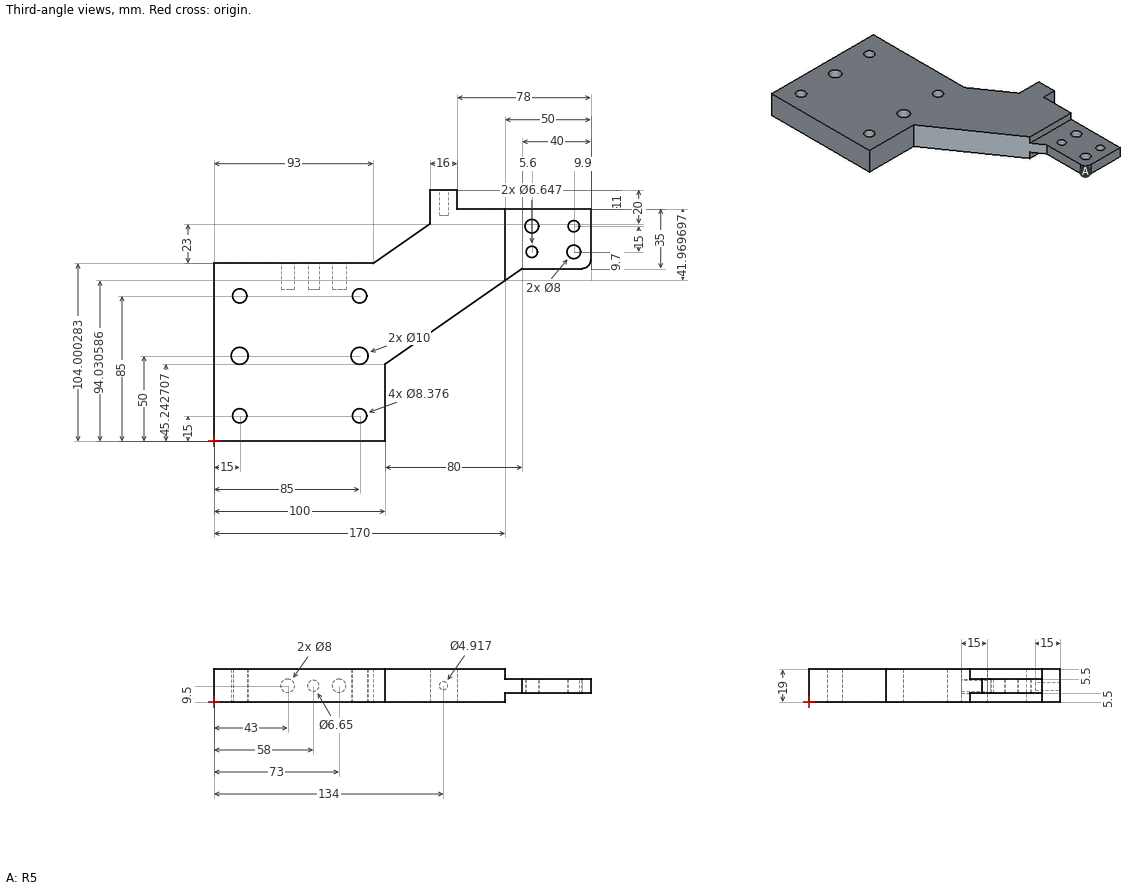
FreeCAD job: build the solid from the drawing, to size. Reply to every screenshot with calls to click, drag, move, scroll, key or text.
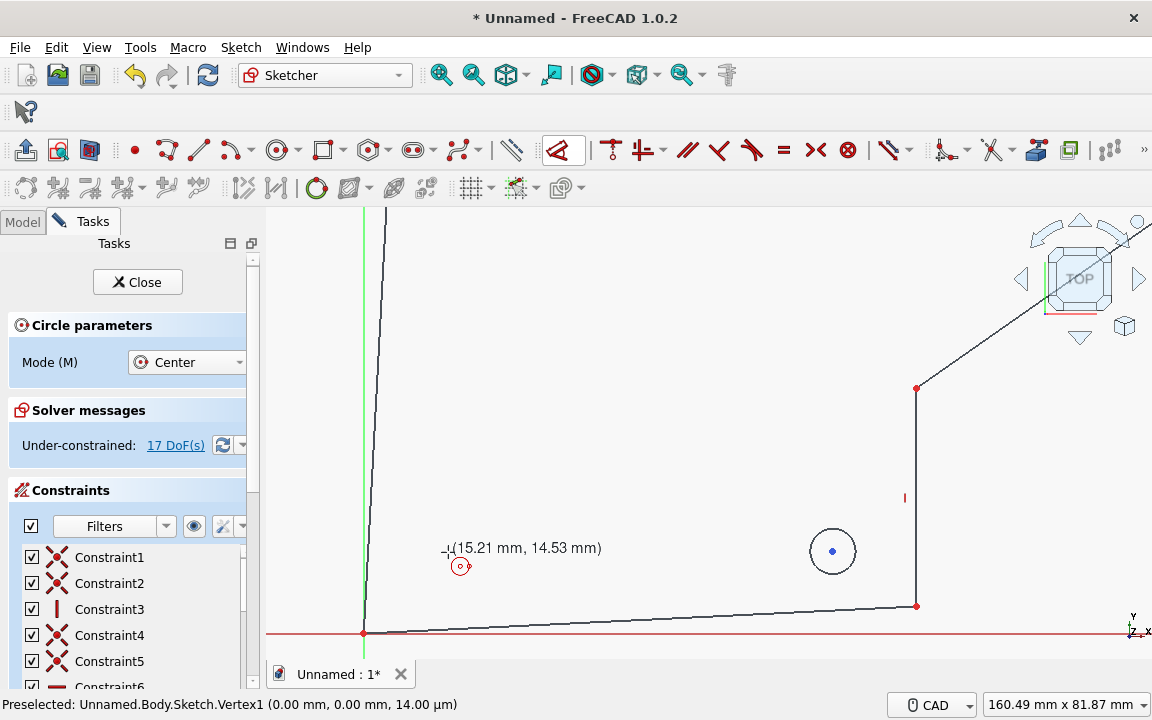
click(447, 551)
click(463, 534)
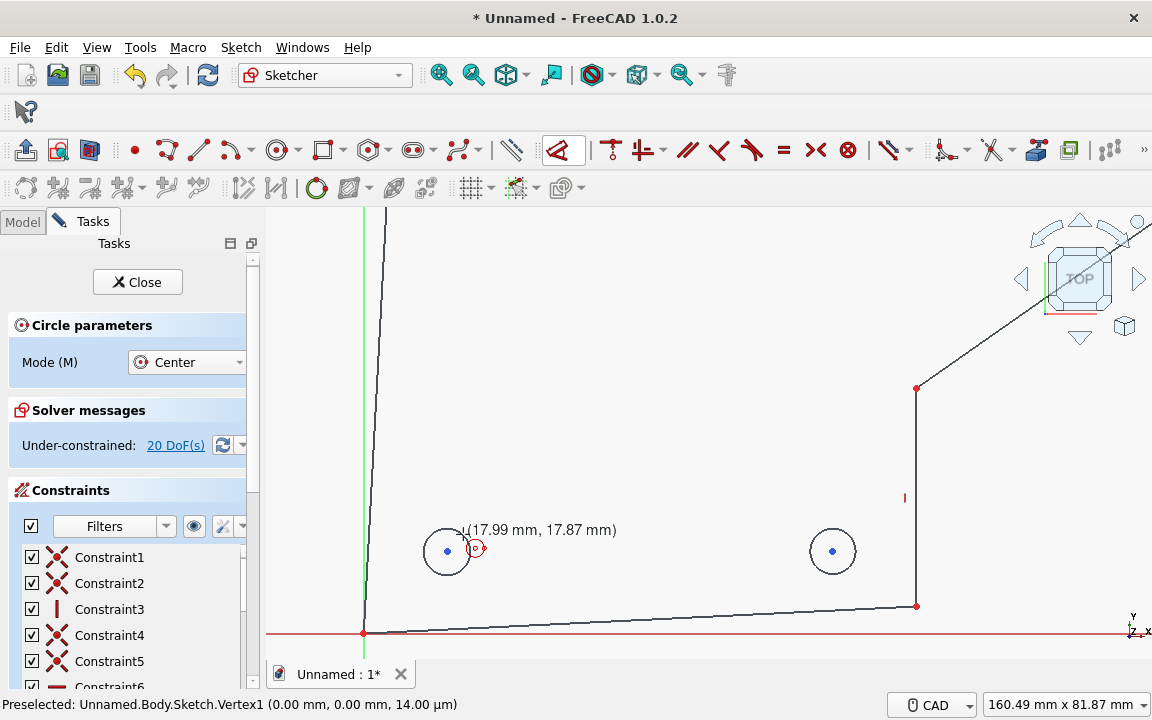
click(833, 358)
click(852, 338)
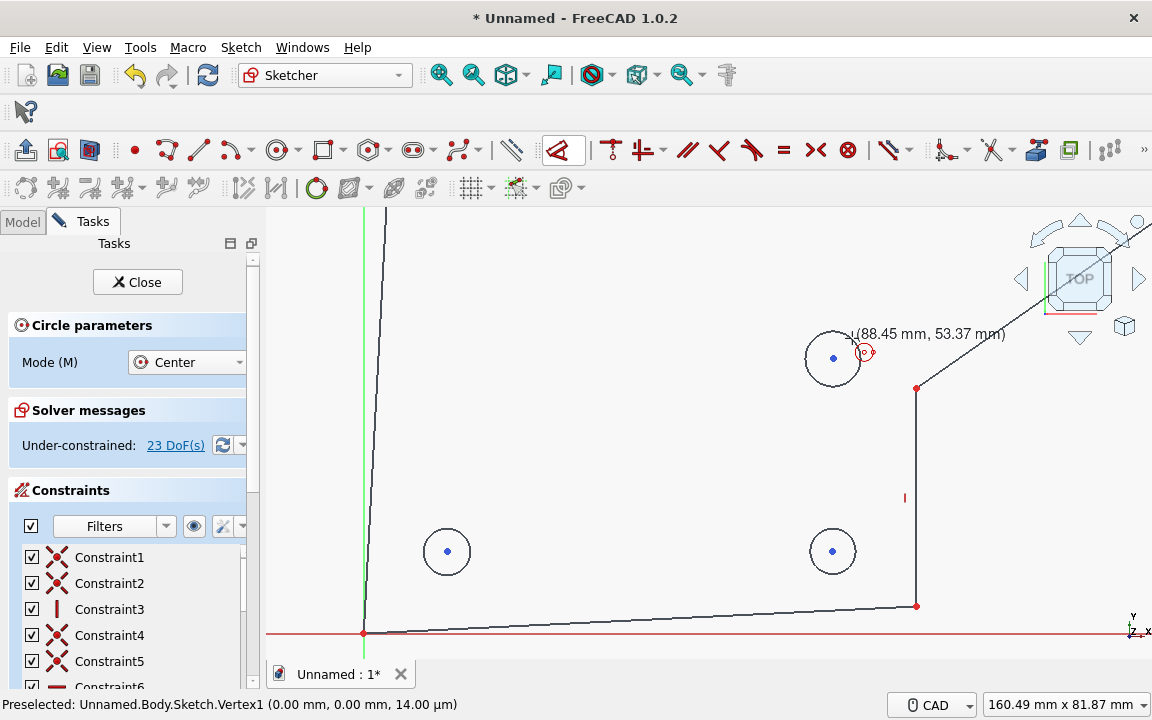
click(447, 358)
click(466, 338)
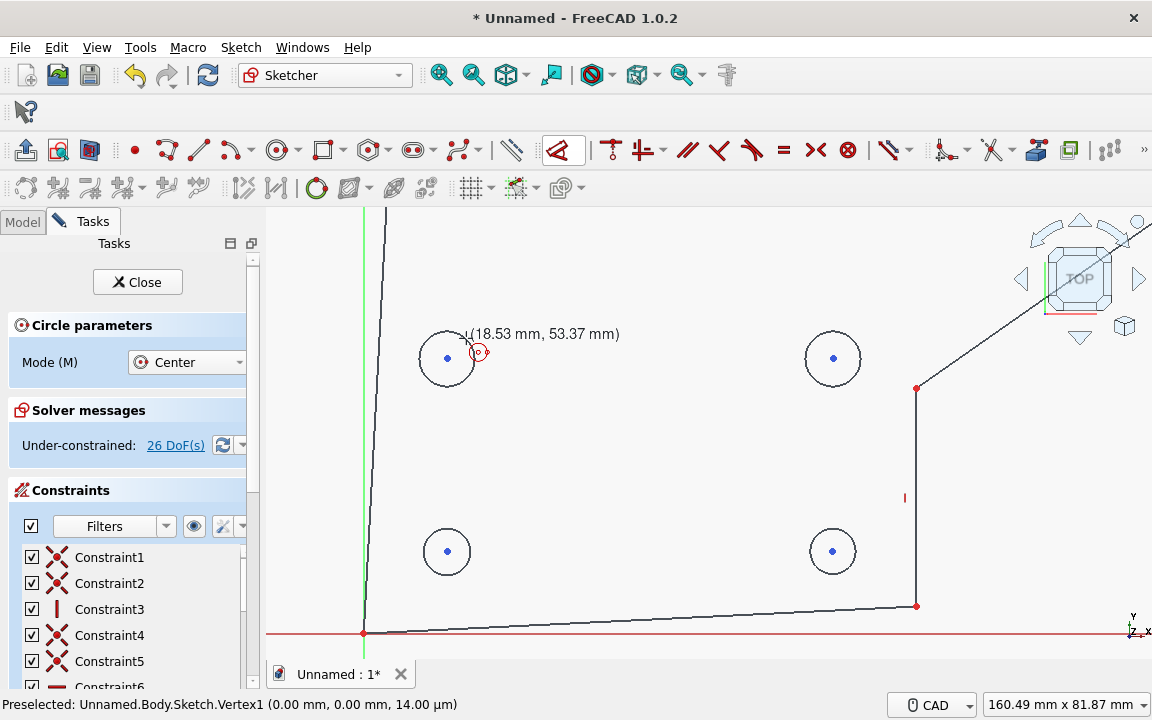
scroll(448, 552, down, 5)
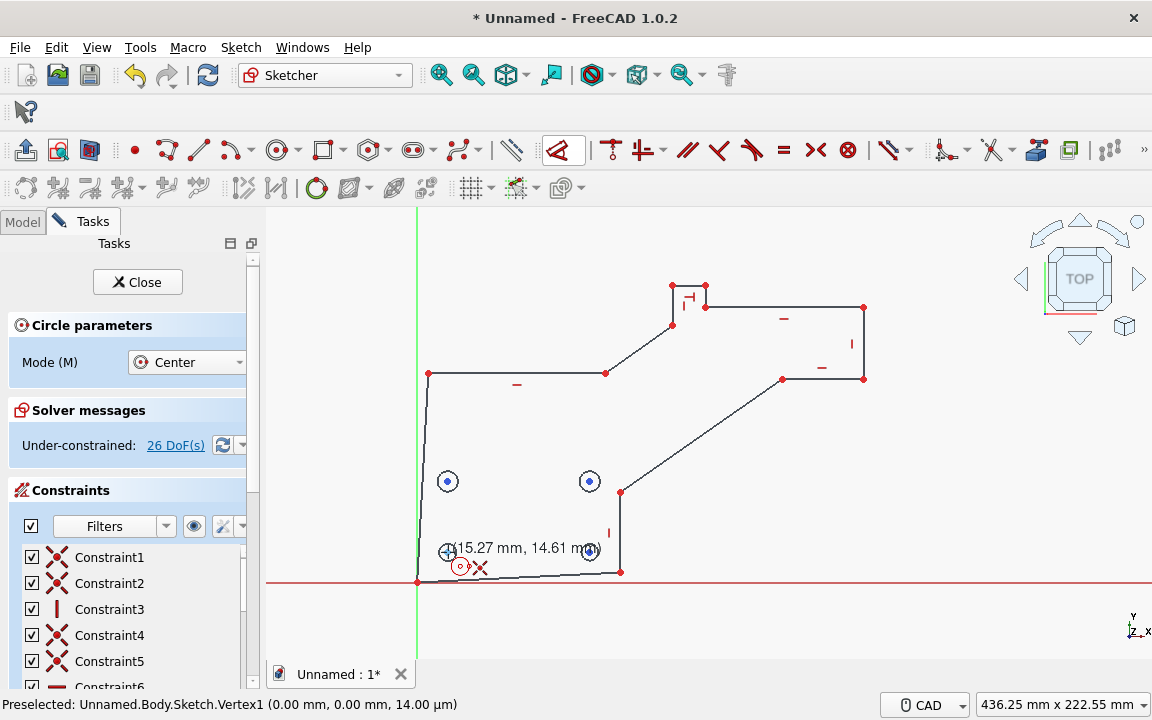
scroll(844, 358, up, 6)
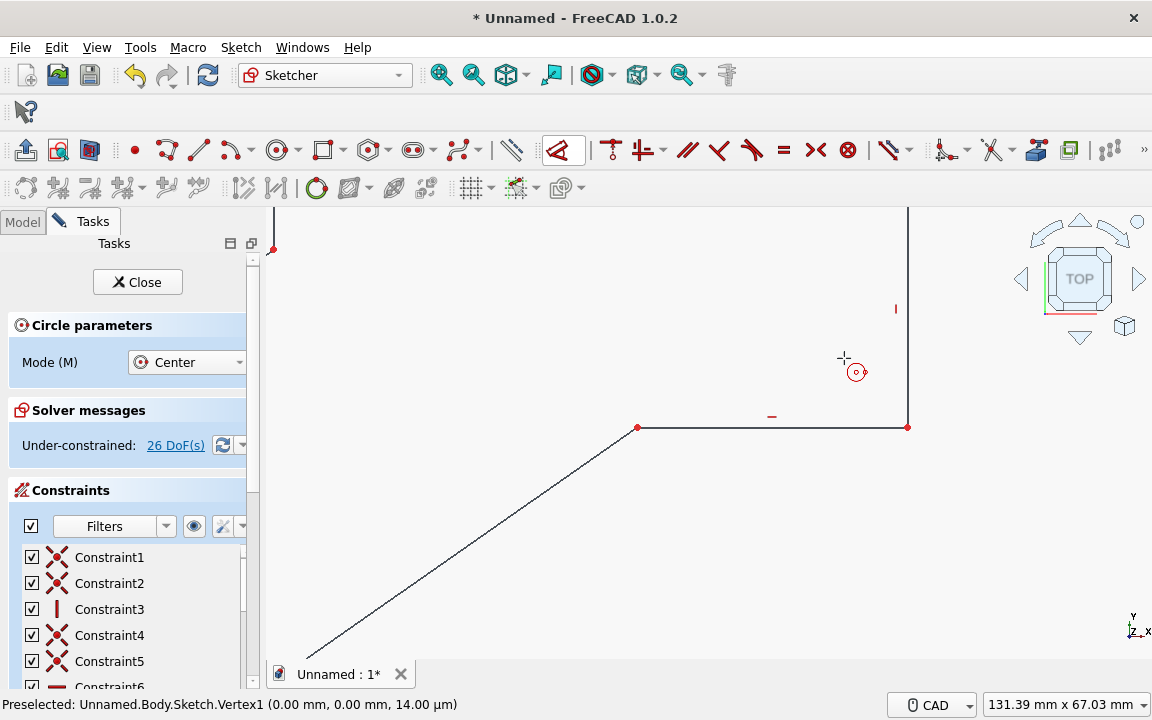
scroll(845, 358, down, 6)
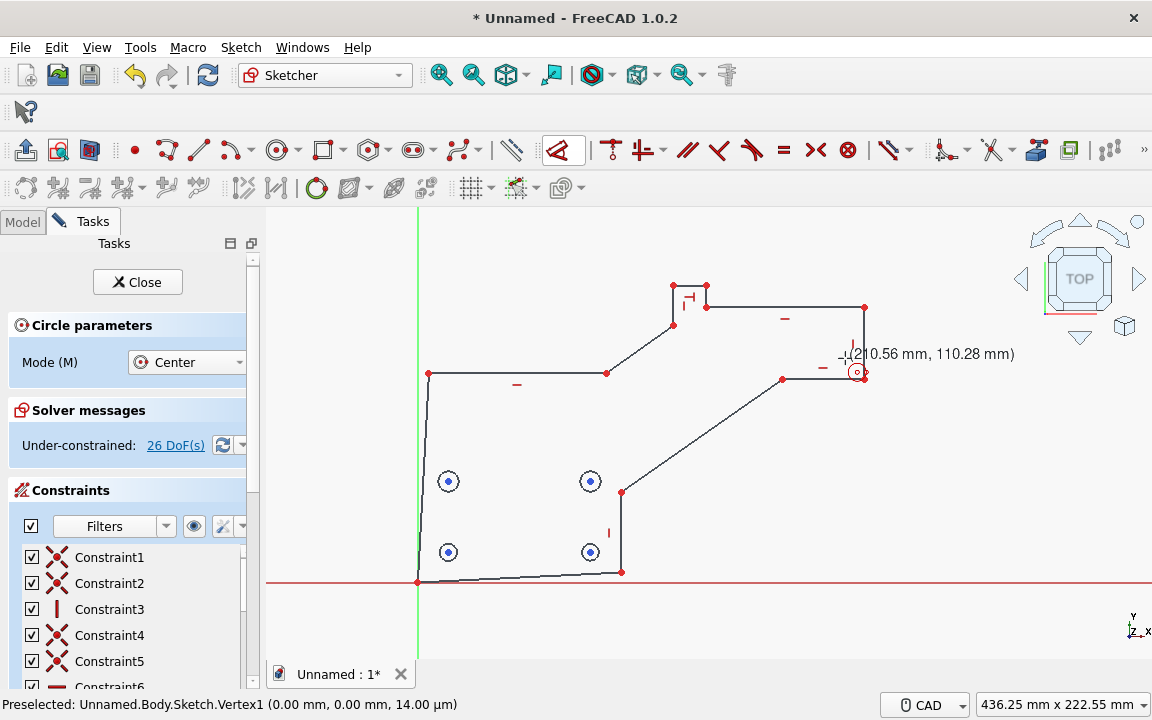
click(845, 358)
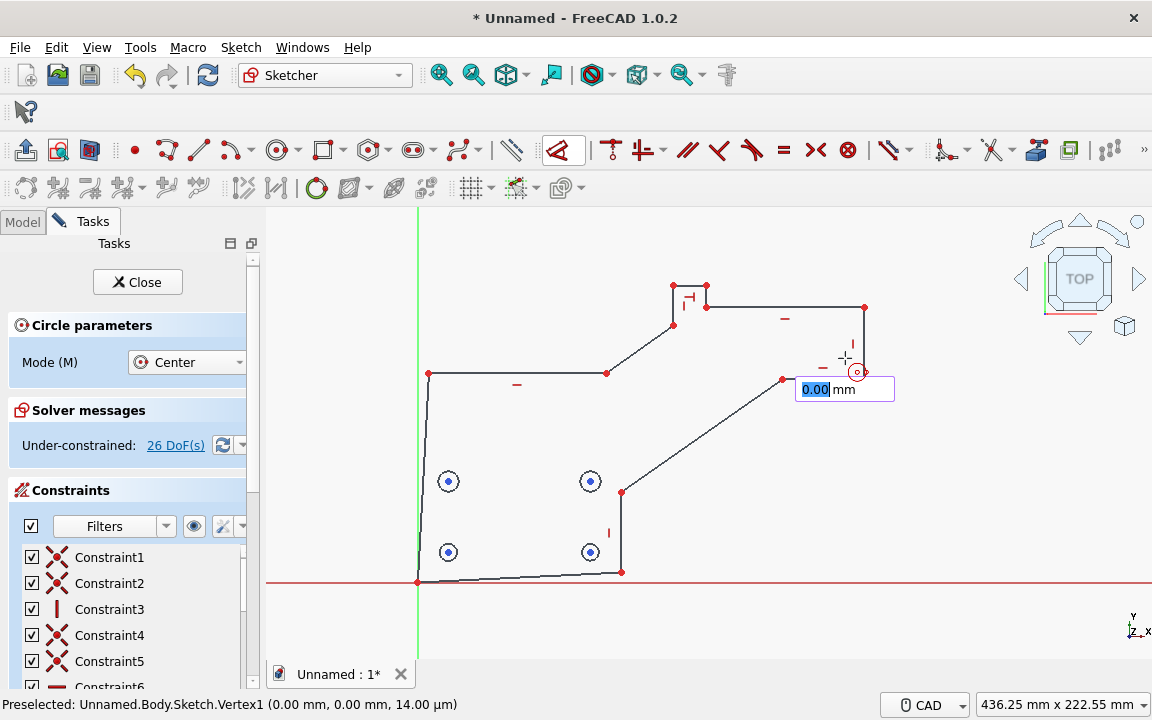
scroll(850, 352, up, 4)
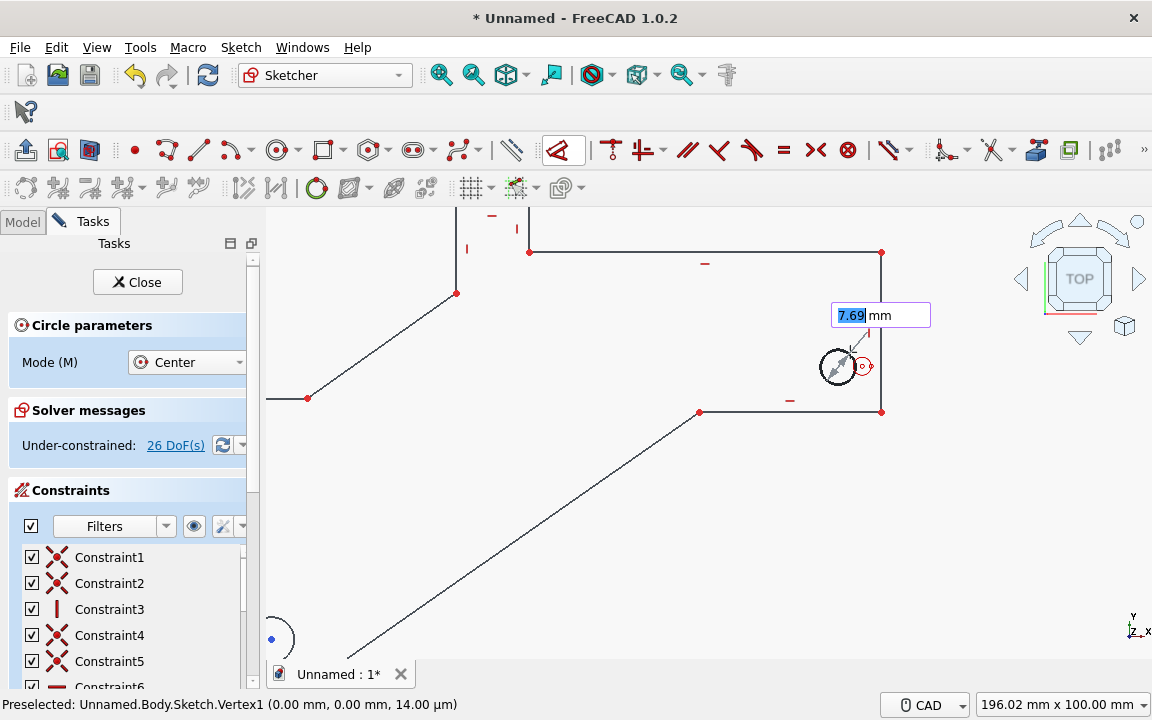
click(850, 351)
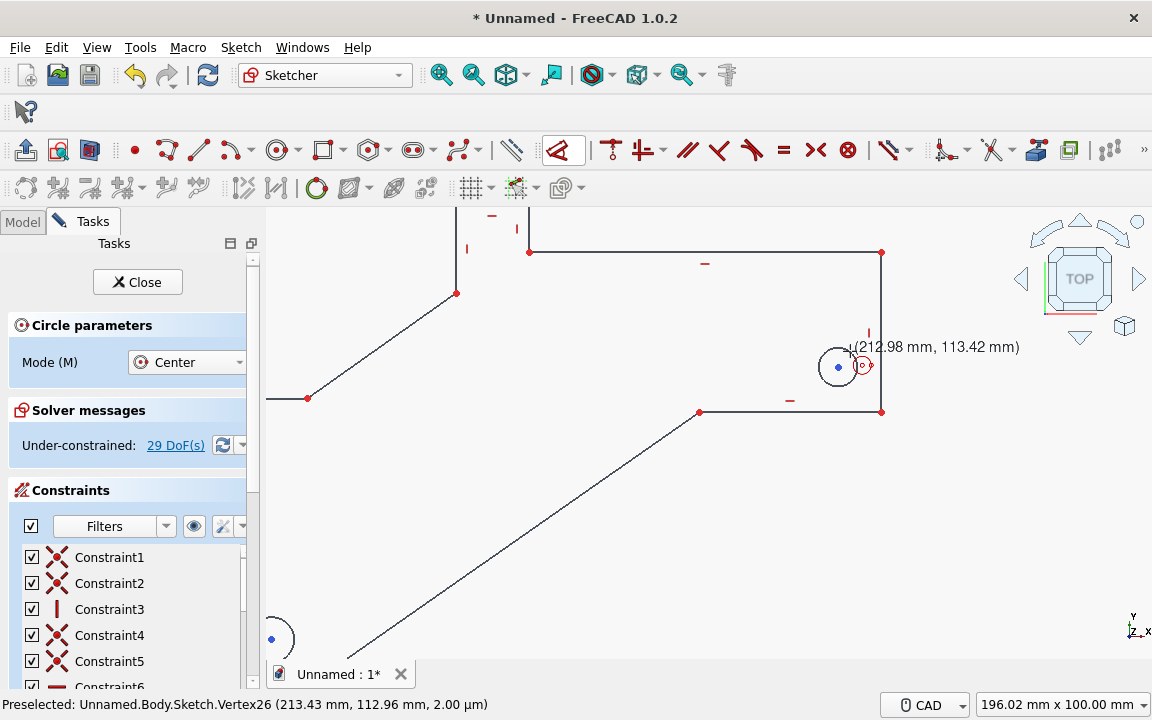
scroll(726, 364, up, 3)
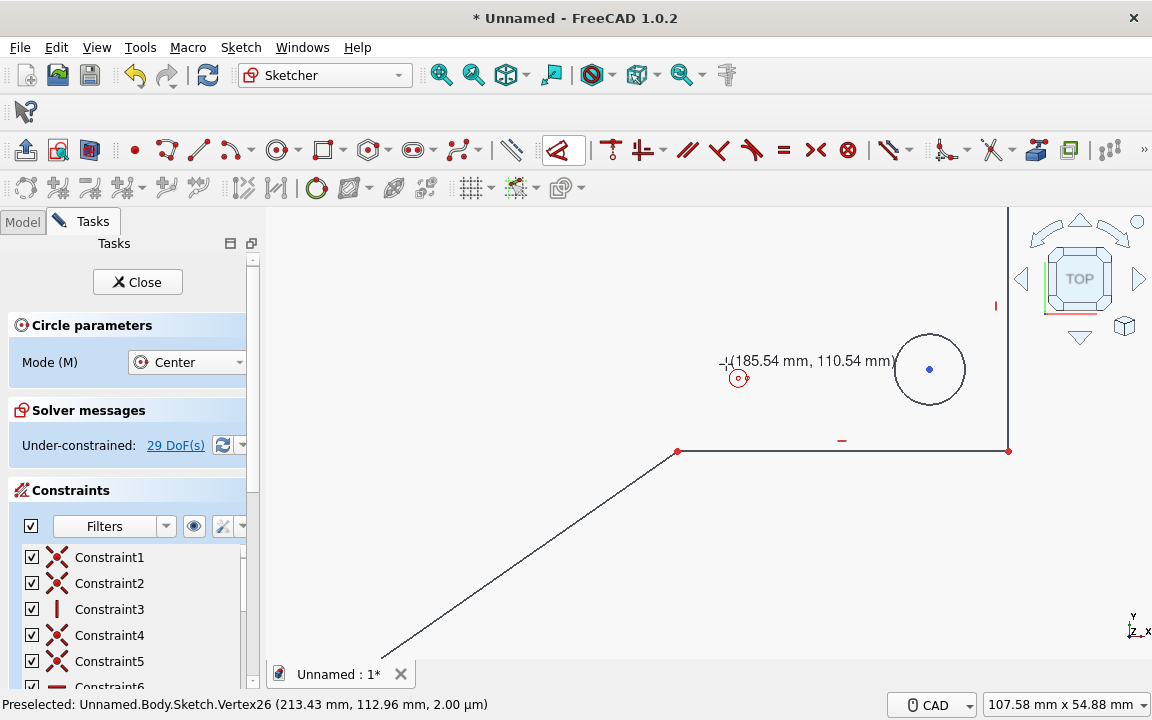
scroll(816, 355, down, 7)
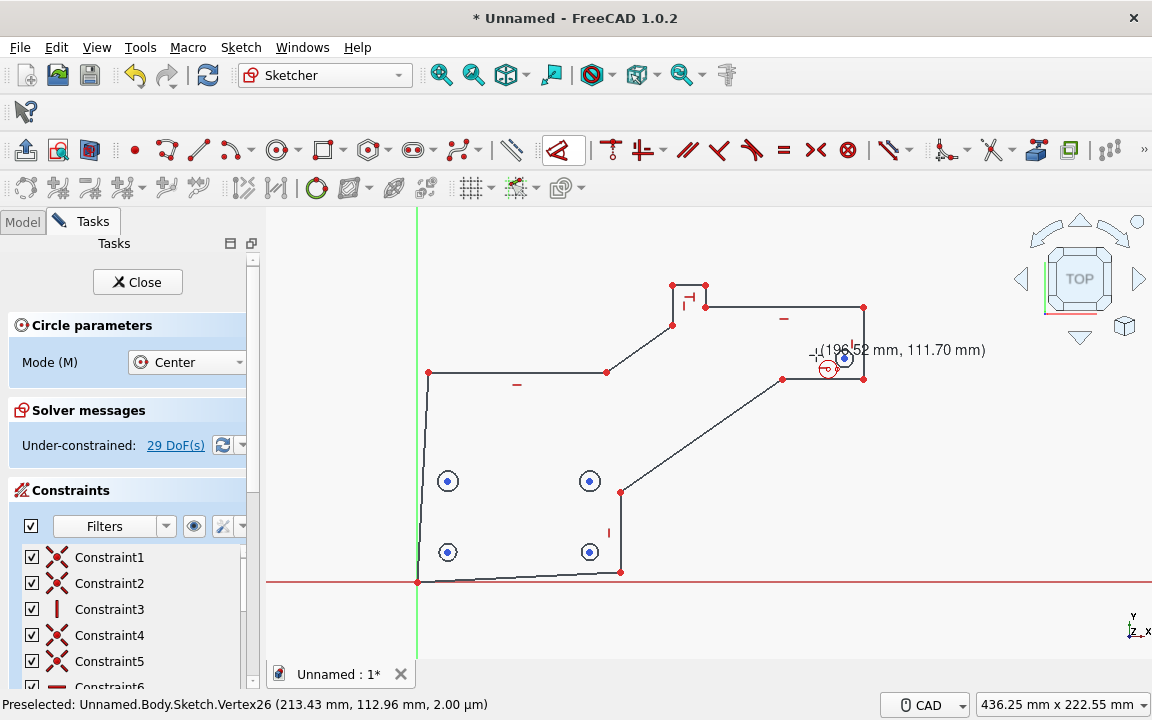
click(794, 358)